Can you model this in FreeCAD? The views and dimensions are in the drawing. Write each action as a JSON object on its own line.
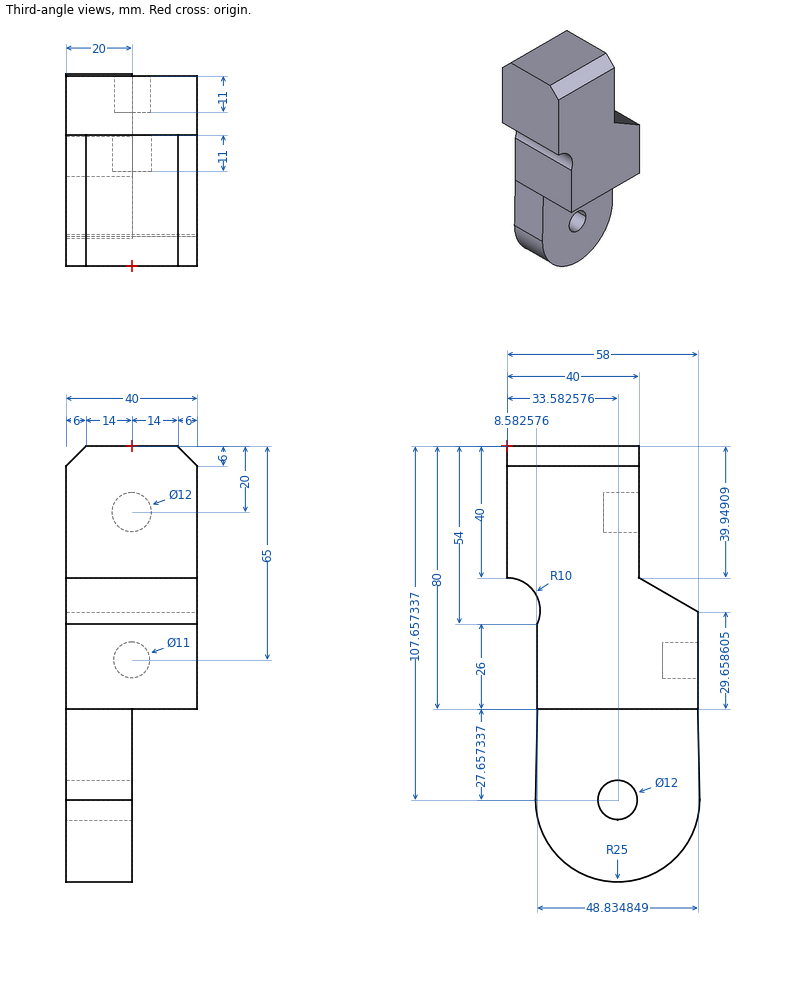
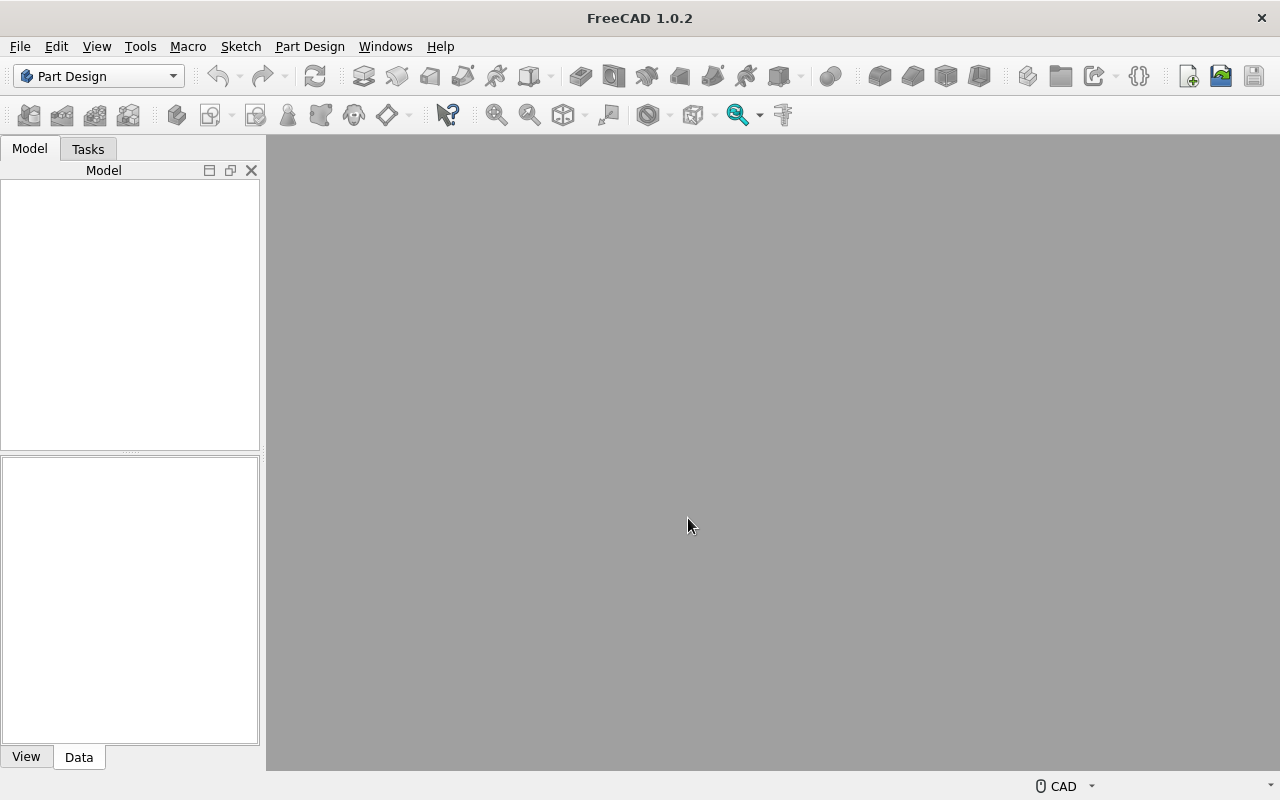
{"action": "left_click", "coordinate": [1188, 76]}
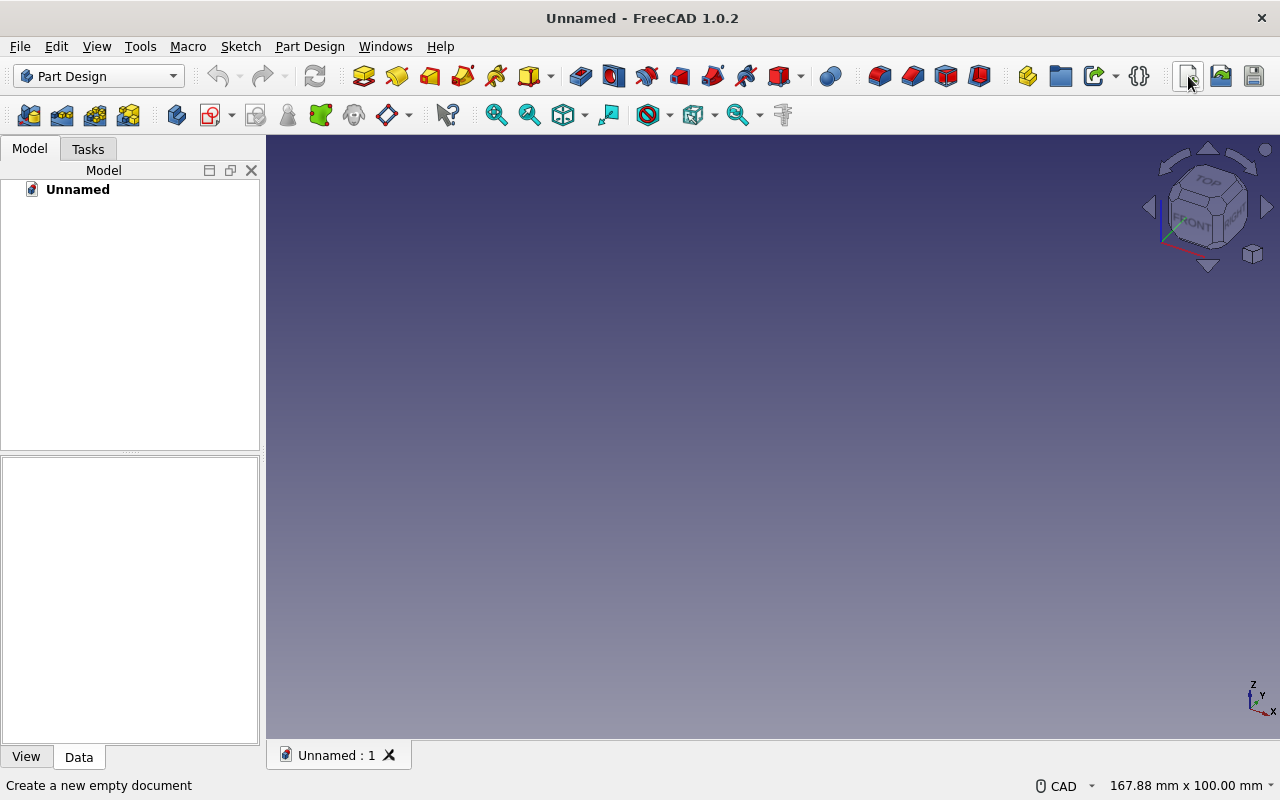
{"action": "left_click", "coordinate": [210, 116]}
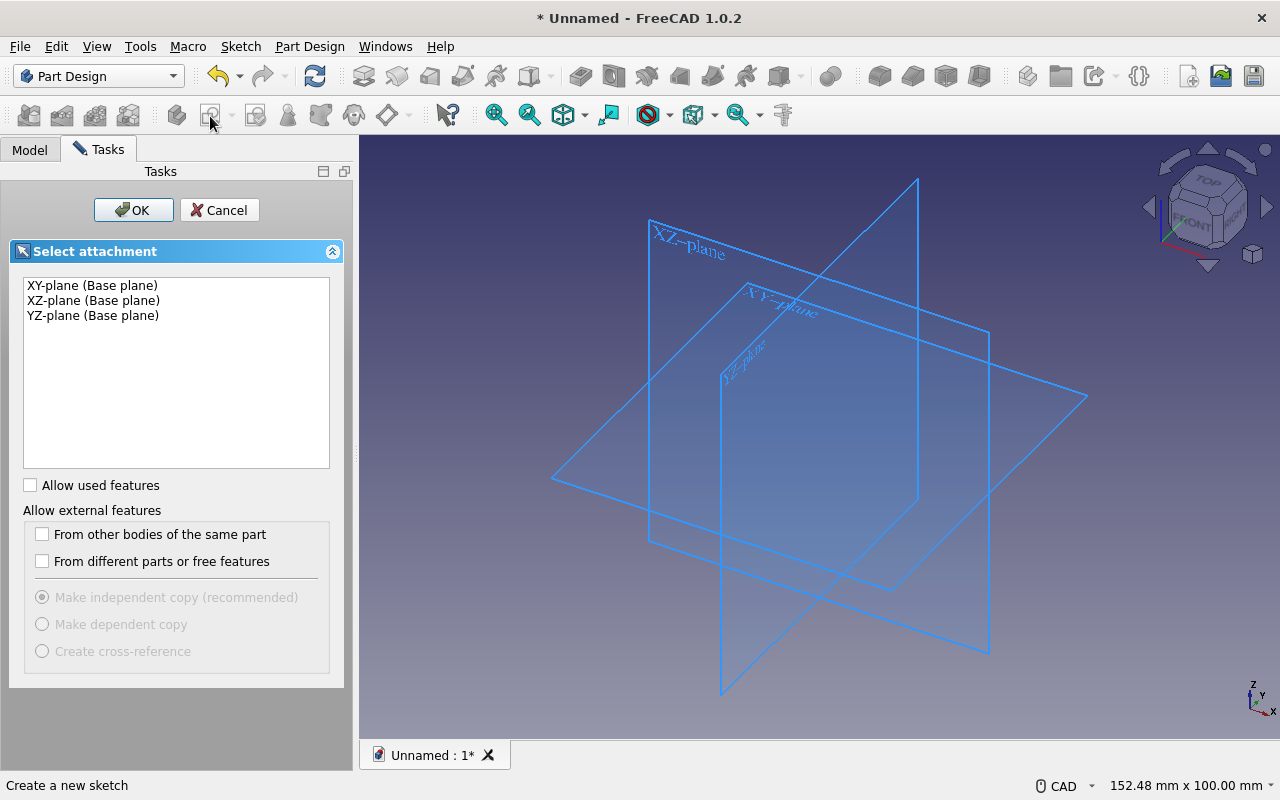
{"action": "left_click", "coordinate": [84, 316]}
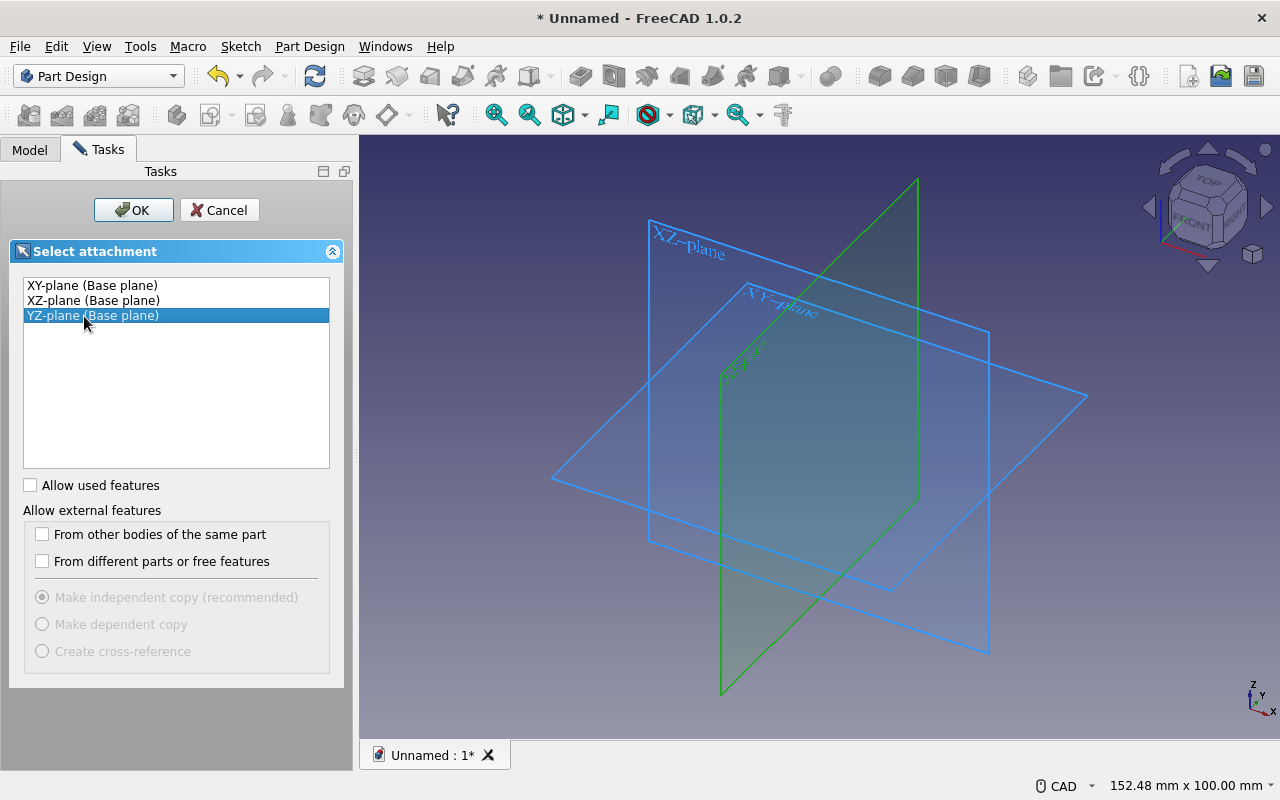
{"action": "left_click", "coordinate": [134, 210]}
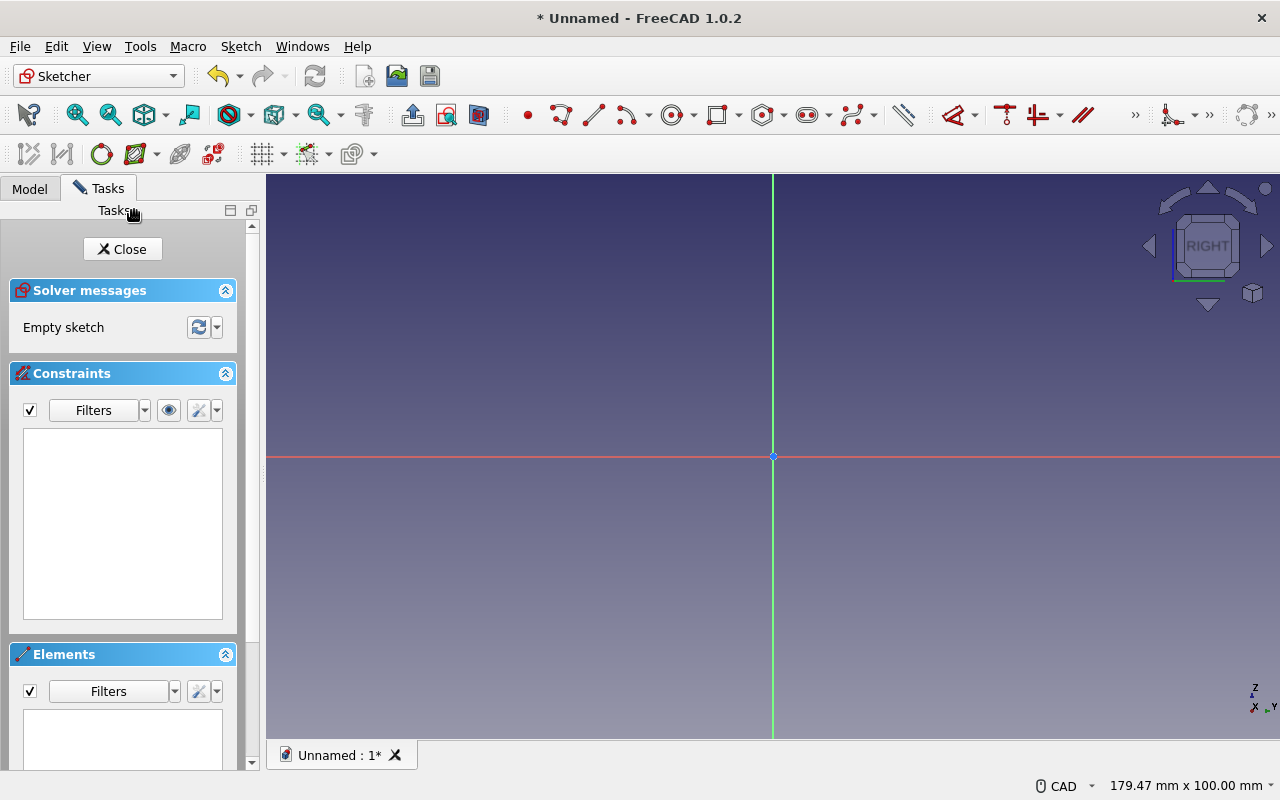
{"action": "scroll", "coordinate": [294, 202], "scroll_direction": "down", "scroll_amount": 2}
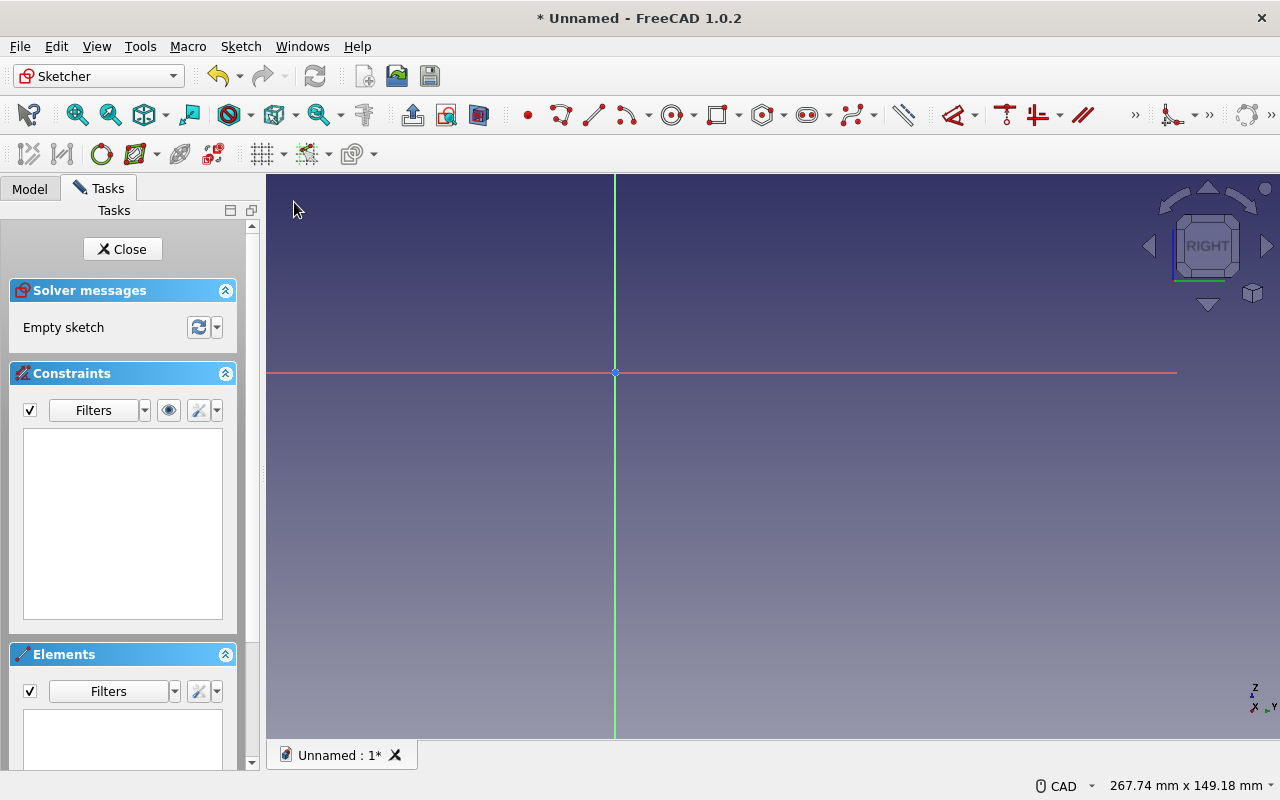
{"action": "left_click", "coordinate": [561, 116]}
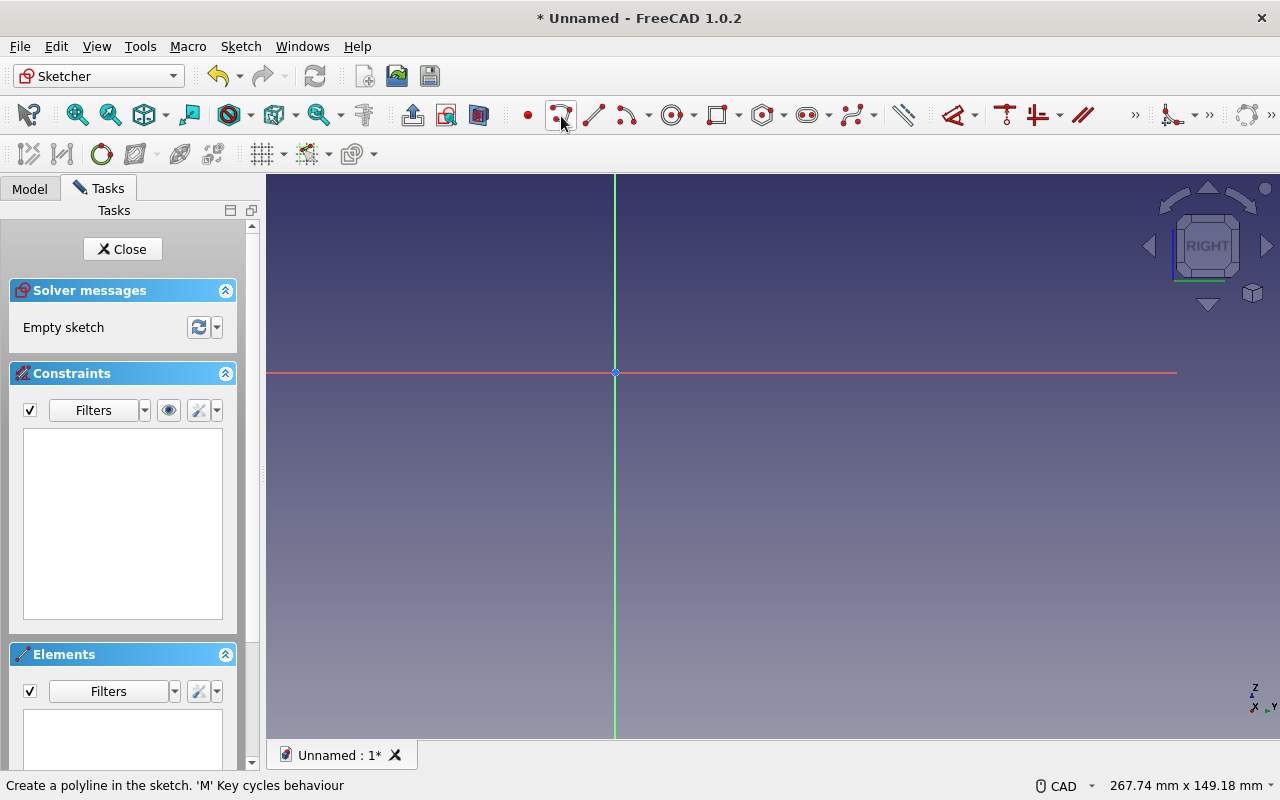
{"action": "left_click", "coordinate": [650, 577]}
{"action": "left_click", "coordinate": [650, 676]}
{"action": "left_click", "coordinate": [835, 676]}
{"action": "left_click", "coordinate": [835, 563]}
{"action": "left_click", "coordinate": [767, 524]}
{"action": "left_click", "coordinate": [767, 373]}
{"action": "left_click", "coordinate": [615, 373]}
{"action": "left_click", "coordinate": [624, 524]}
{"action": "right_click", "coordinate": [624, 524]}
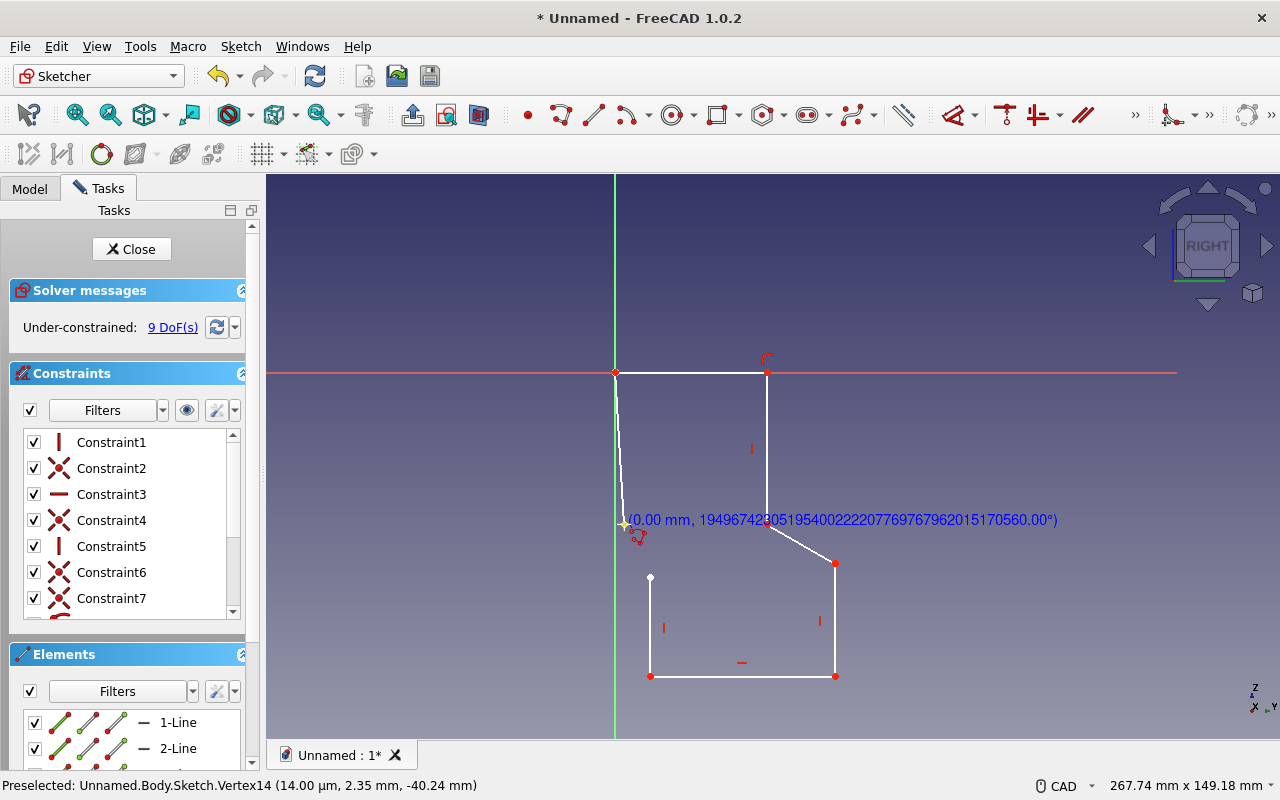
{"action": "key", "text": "g 3 a"}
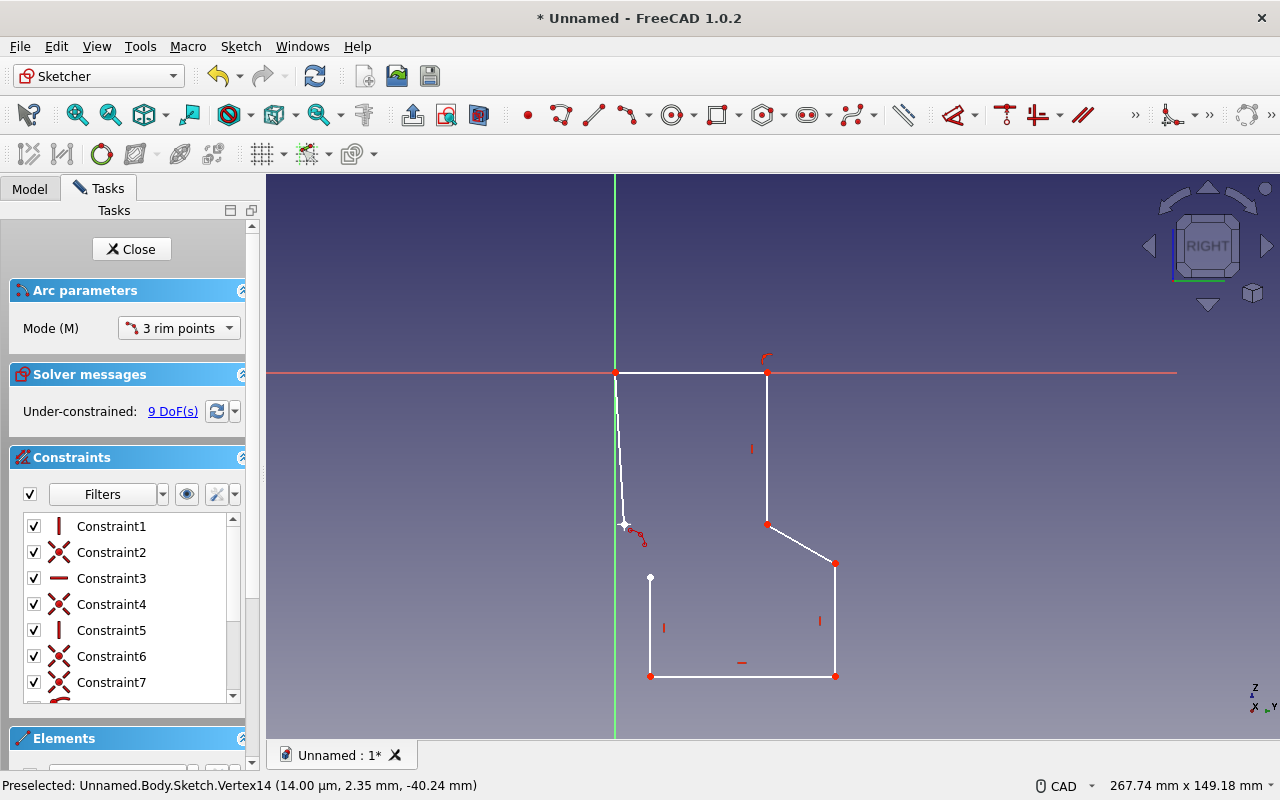
{"action": "left_click", "coordinate": [624, 525]}
{"action": "left_click", "coordinate": [650, 578]}
{"action": "left_click", "coordinate": [647, 541]}
{"action": "key", "text": "Escape"}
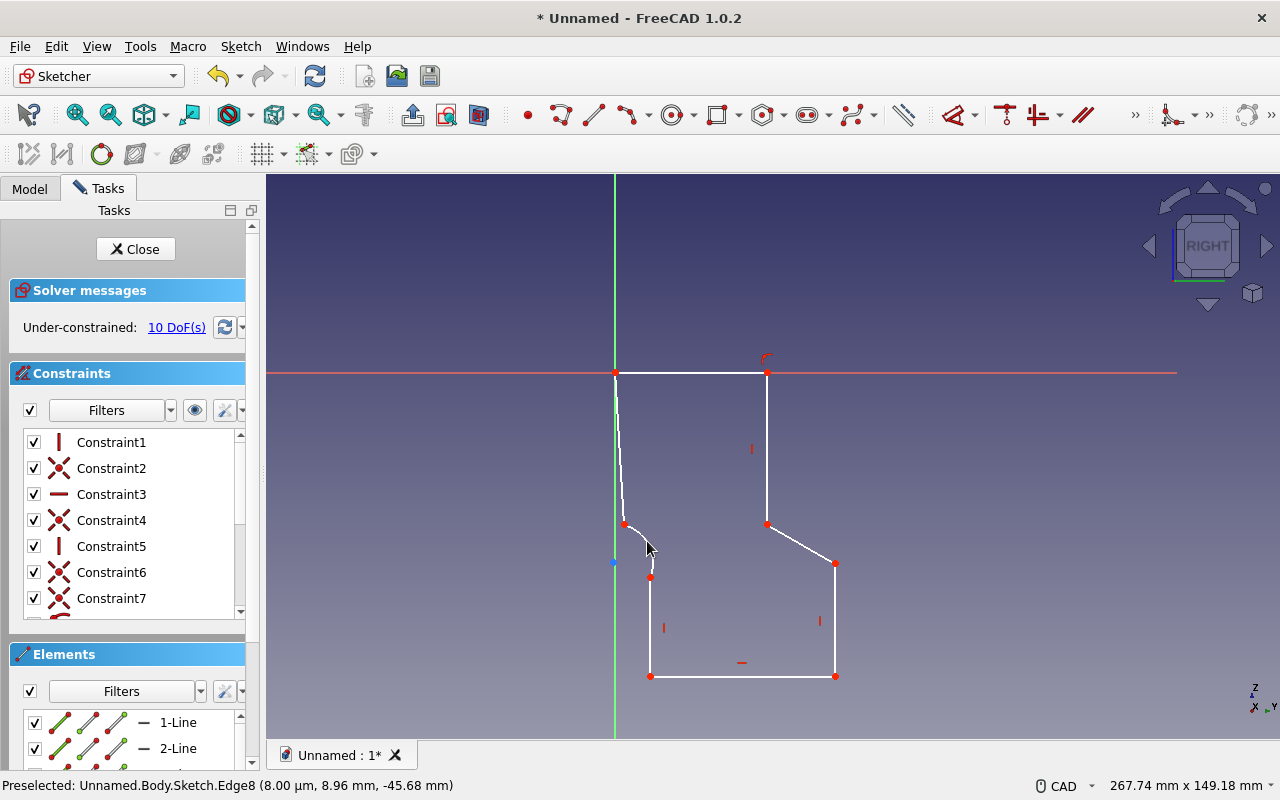
{"action": "left_click", "coordinate": [618, 418]}